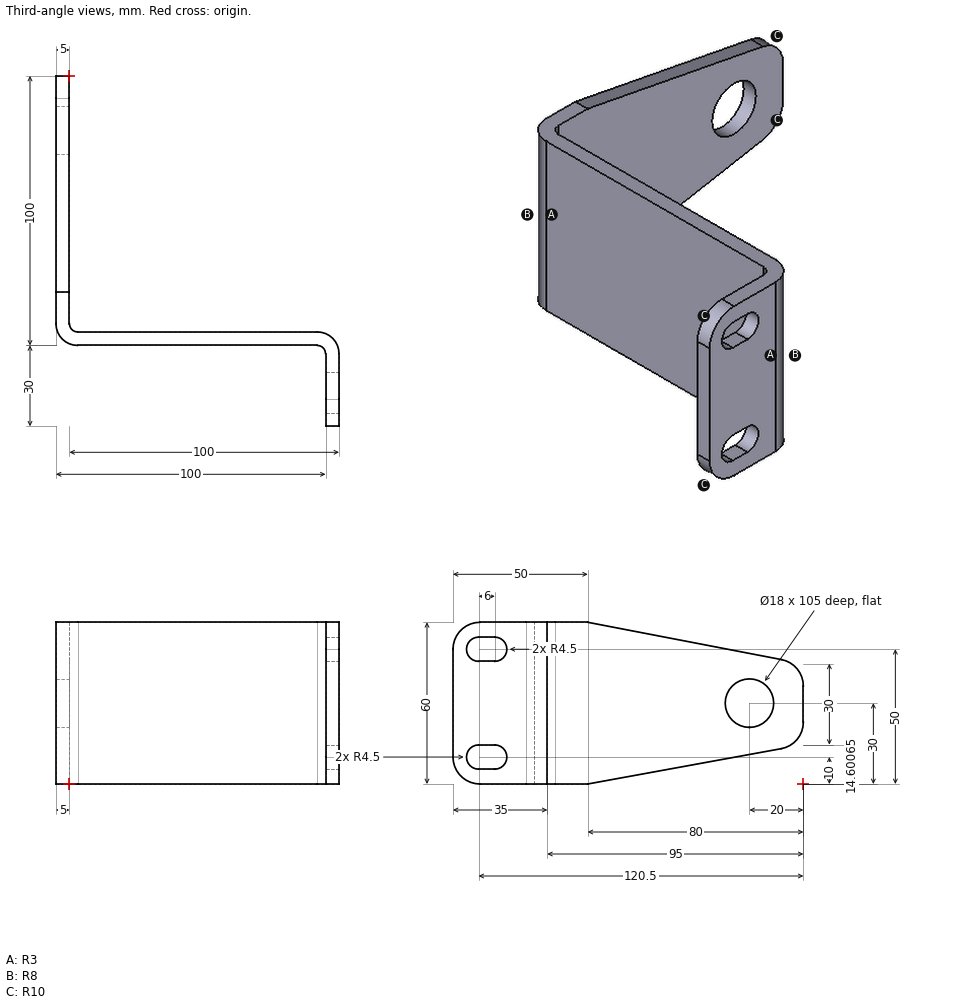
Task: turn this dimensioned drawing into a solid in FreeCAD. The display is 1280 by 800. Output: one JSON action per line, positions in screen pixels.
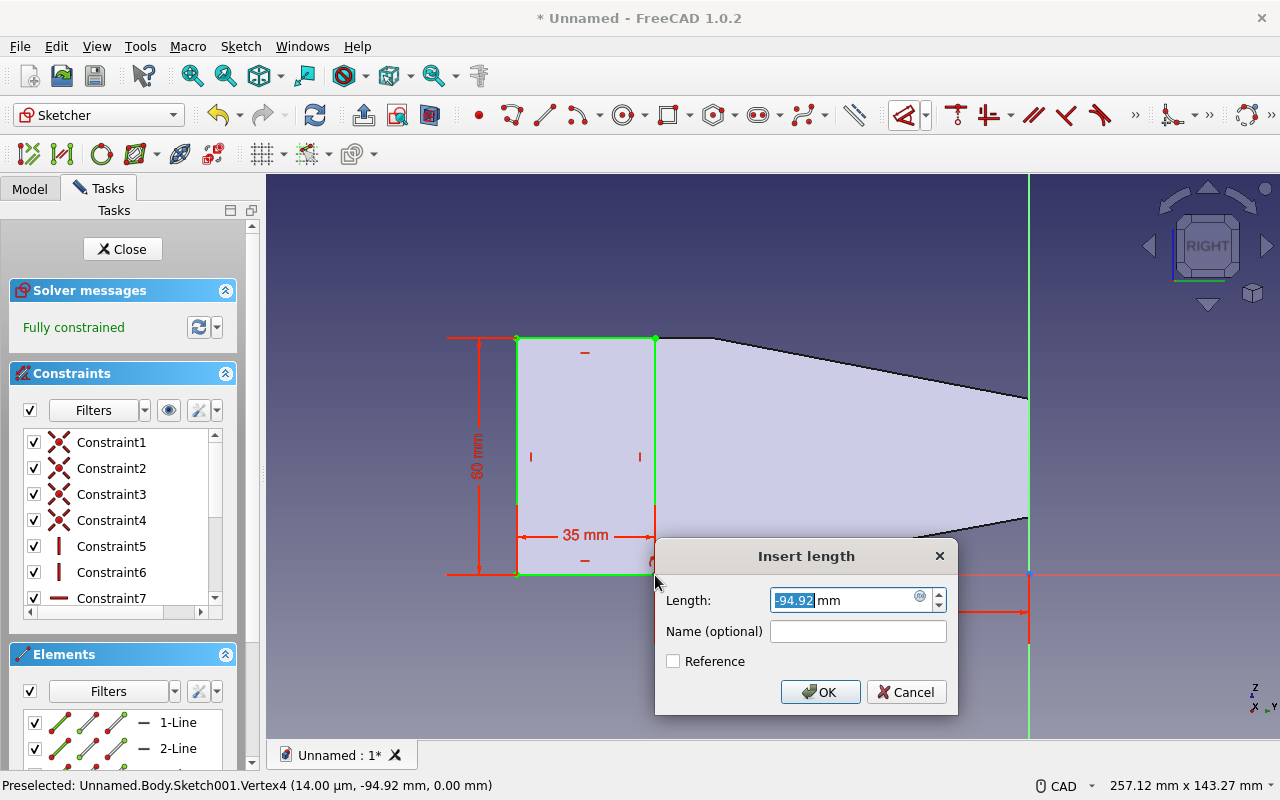
{"action": "type", "text": "-95"}
{"action": "key", "text": "Return"}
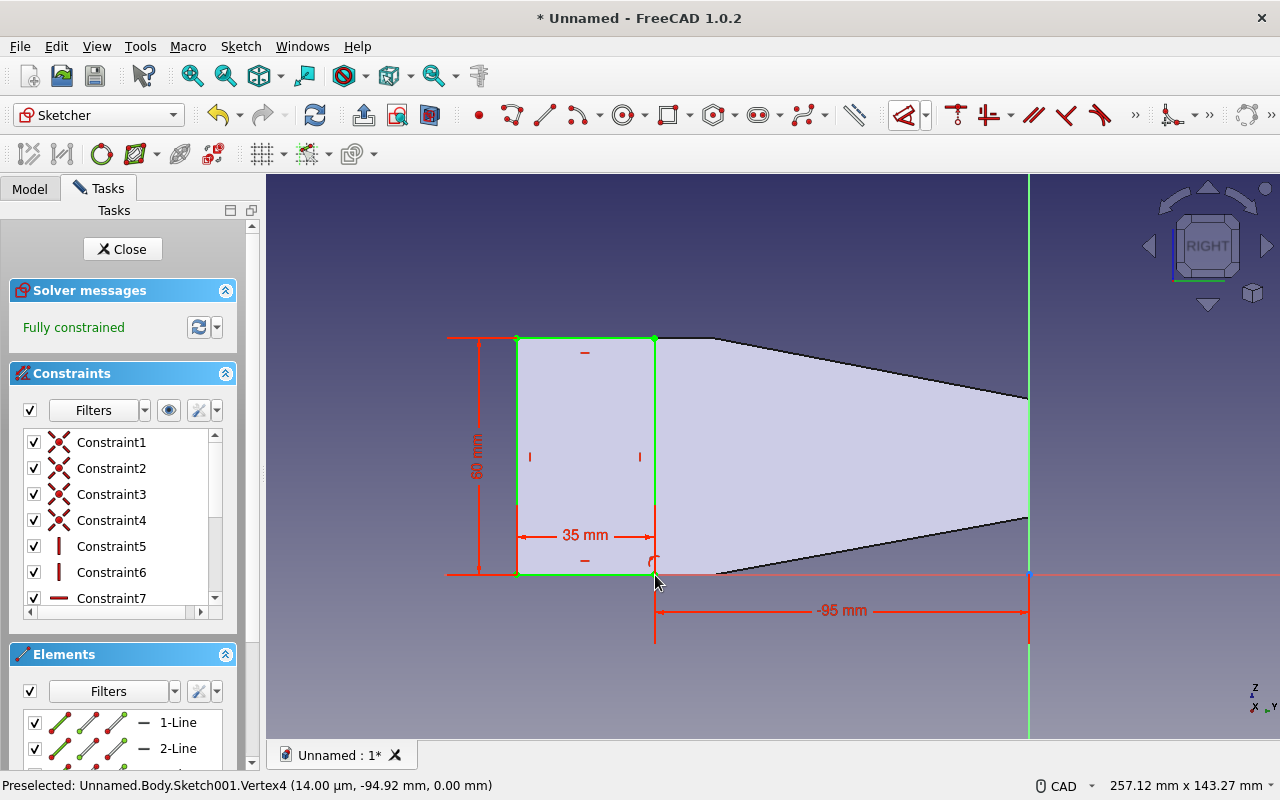
{"action": "left_click", "coordinate": [123, 249]}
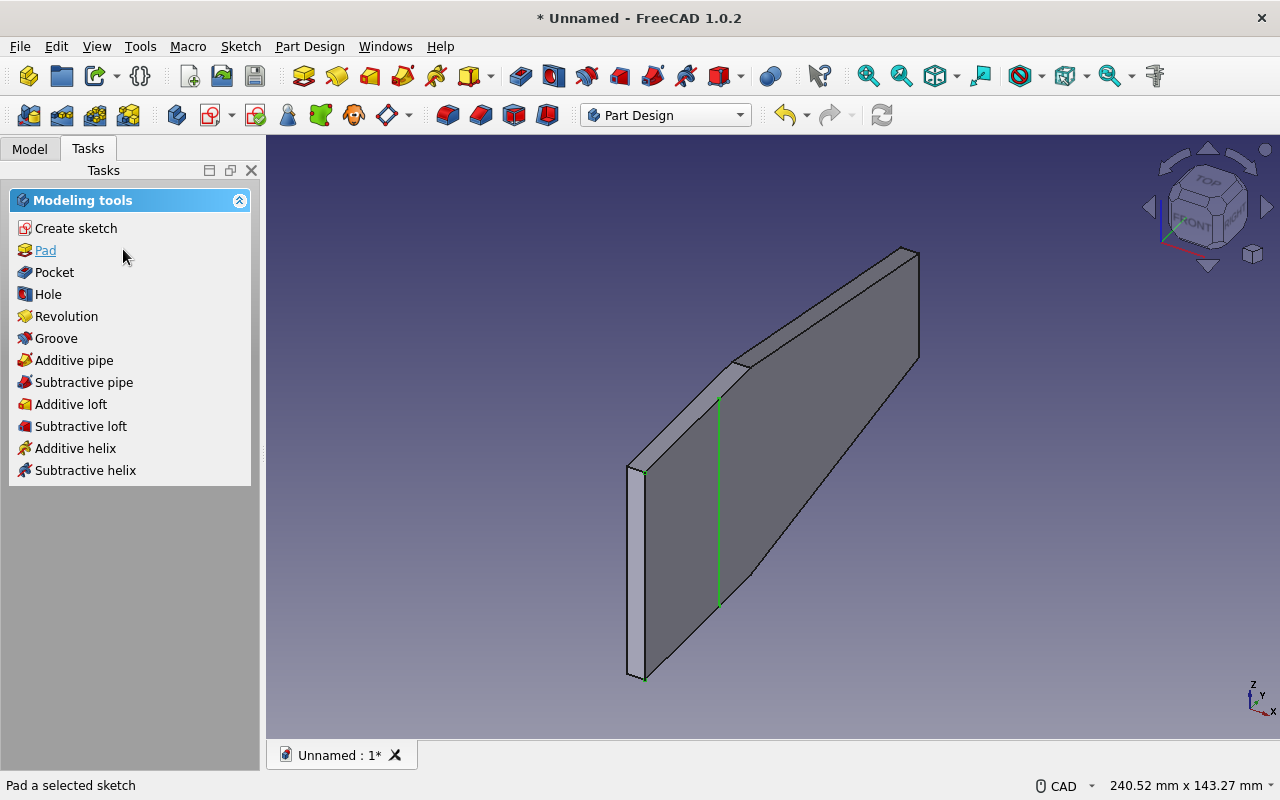
{"action": "left_click", "coordinate": [304, 76]}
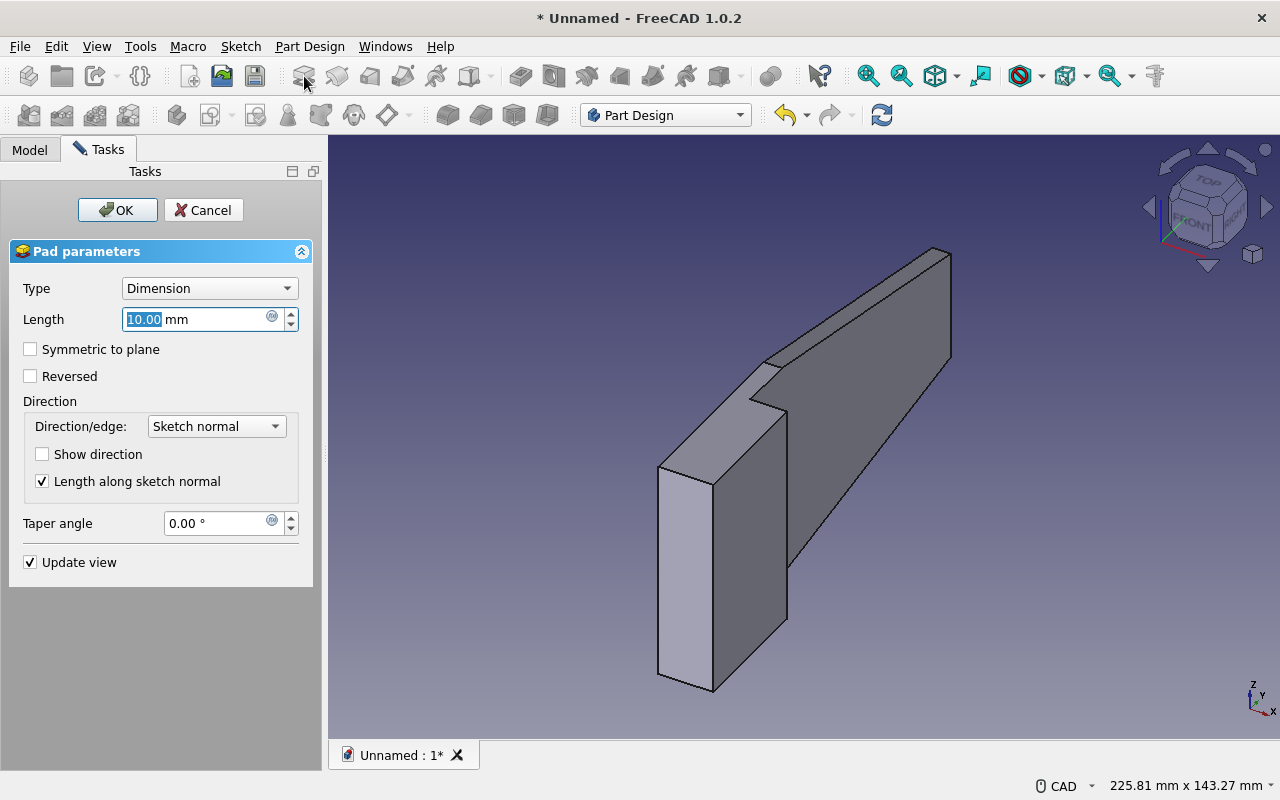
{"action": "type", "text": "100"}
{"action": "key", "text": "Tab"}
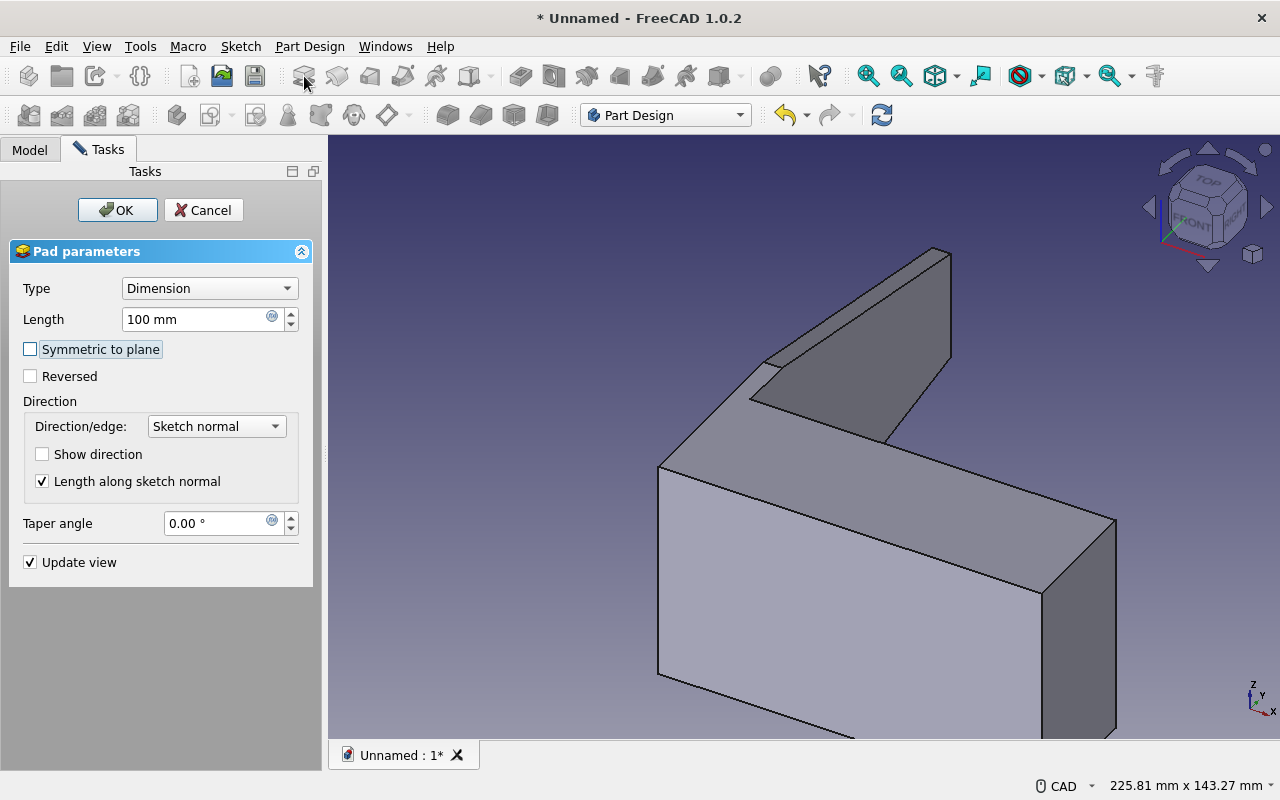
{"action": "left_click", "coordinate": [118, 210]}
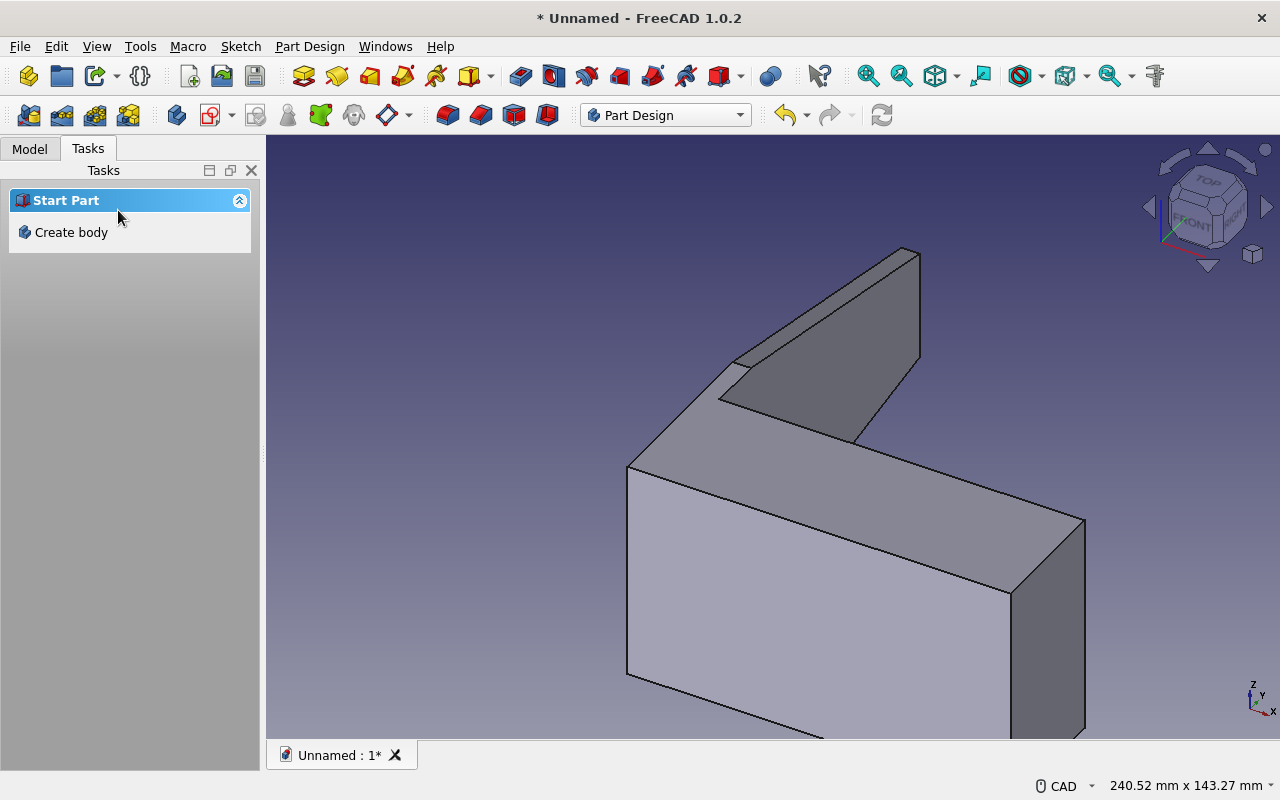
{"action": "left_click", "coordinate": [869, 76]}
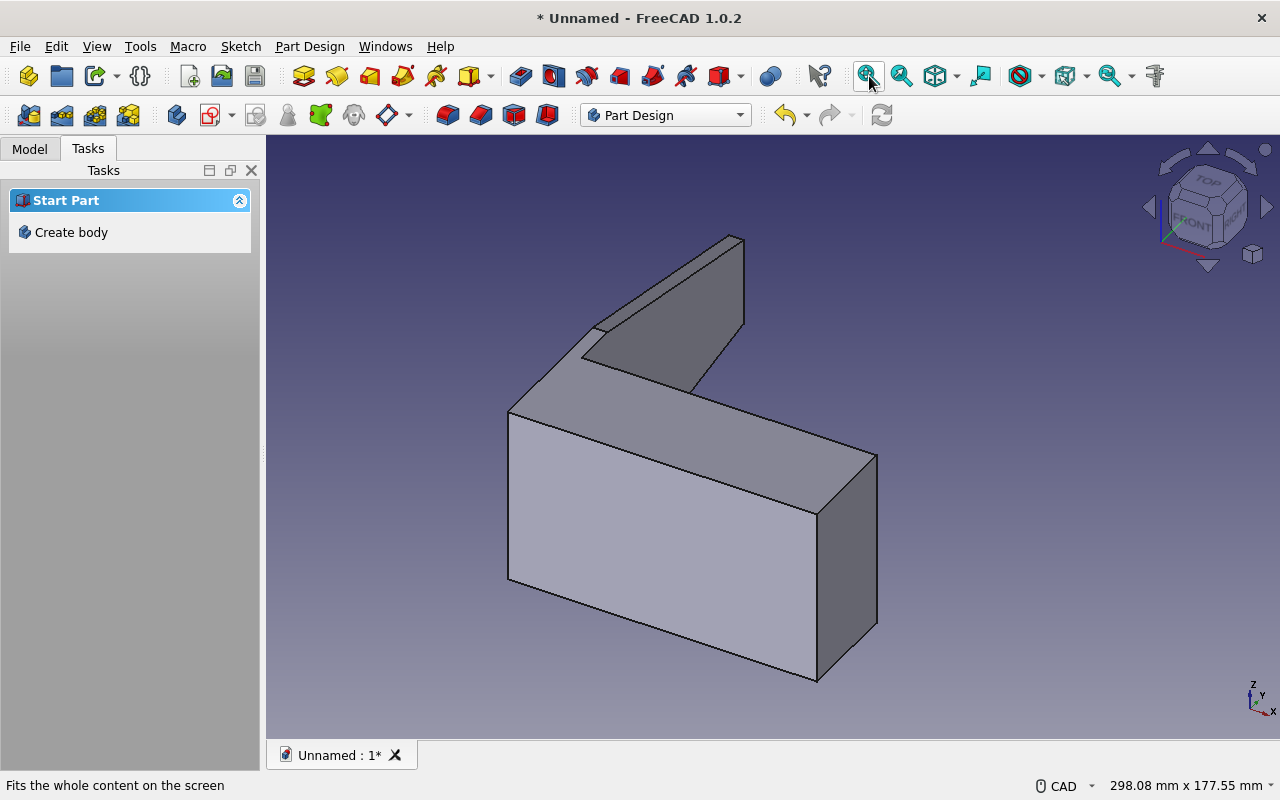
{"action": "left_click", "coordinate": [210, 116]}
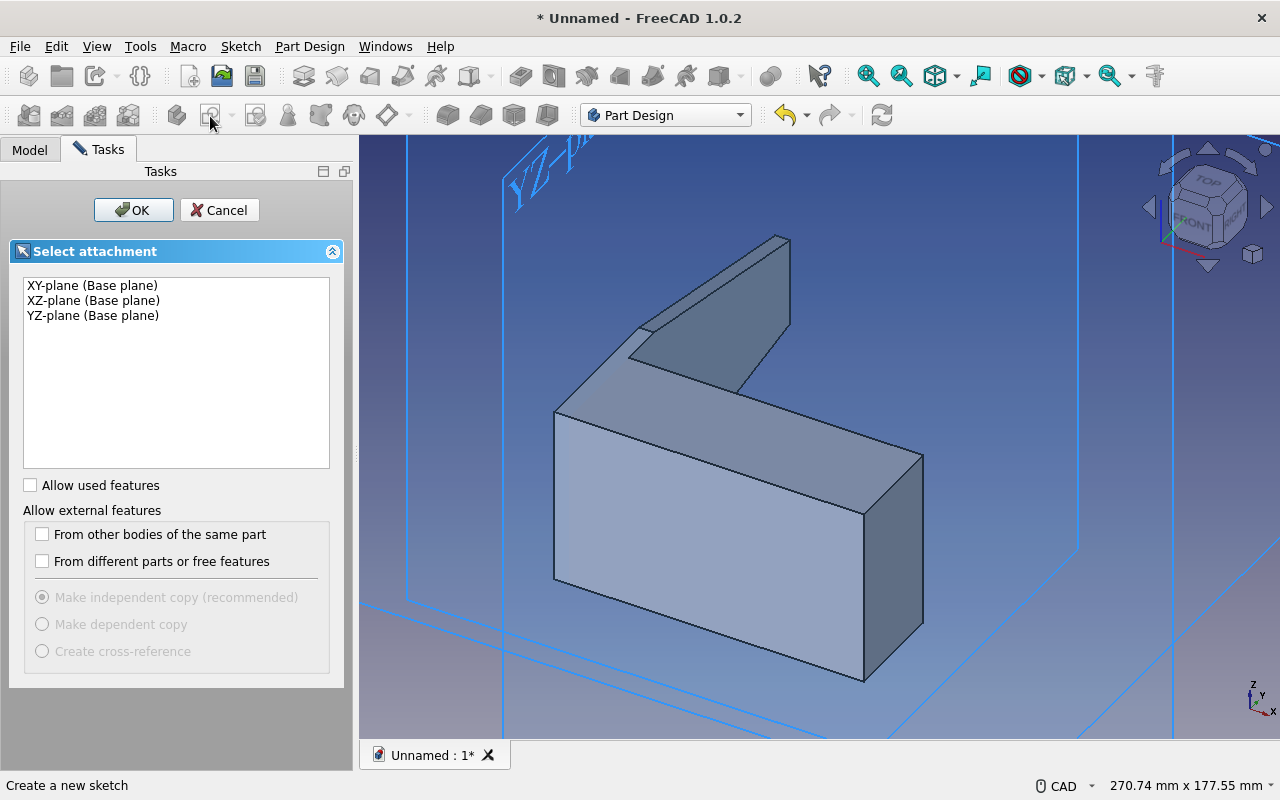
{"action": "left_click", "coordinate": [84, 286]}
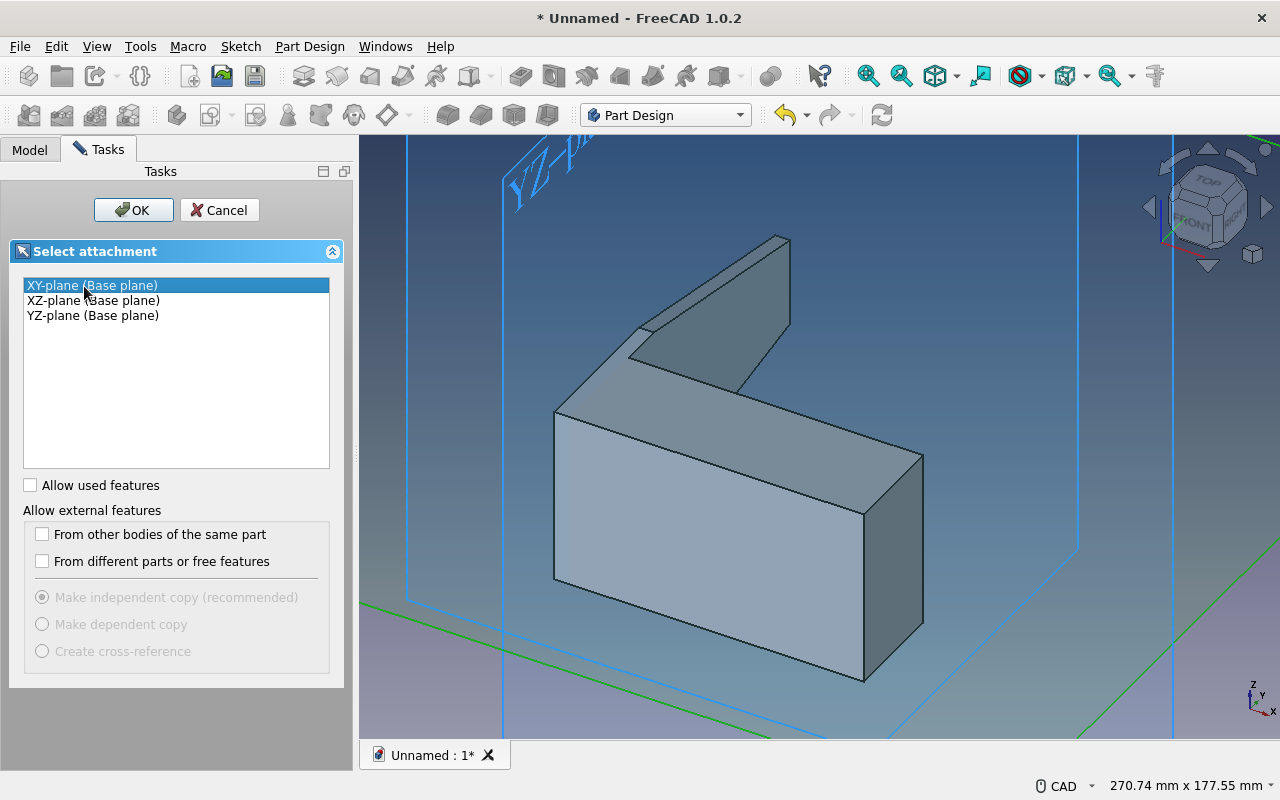
{"action": "left_click", "coordinate": [134, 210]}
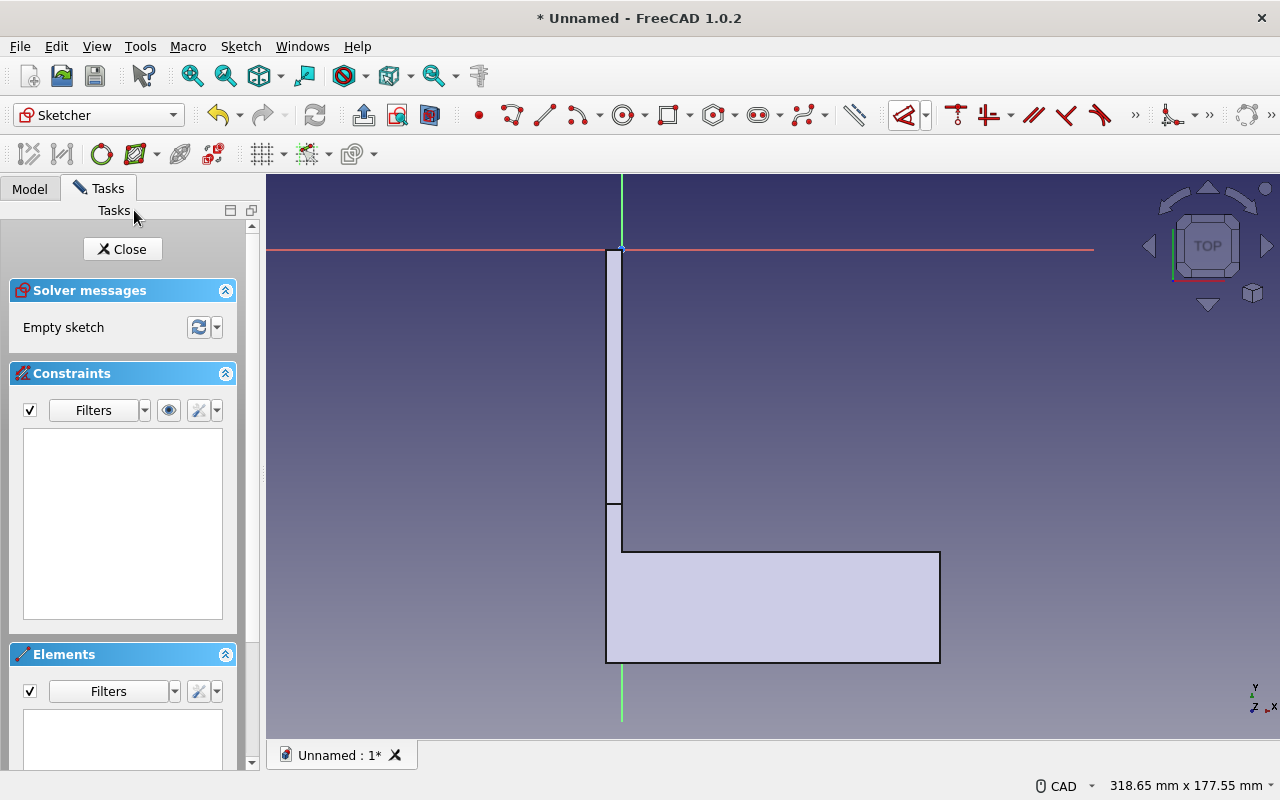
{"action": "left_click", "coordinate": [430, 116]}